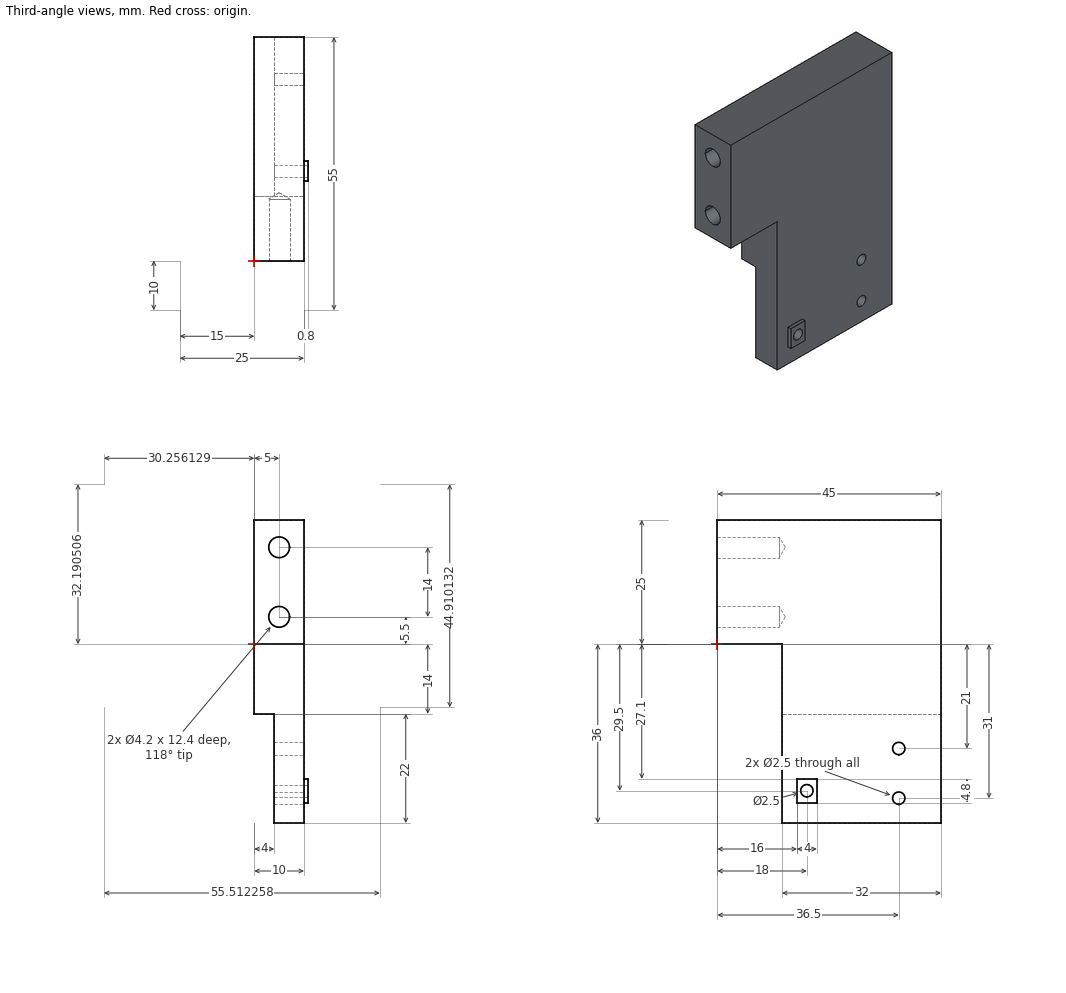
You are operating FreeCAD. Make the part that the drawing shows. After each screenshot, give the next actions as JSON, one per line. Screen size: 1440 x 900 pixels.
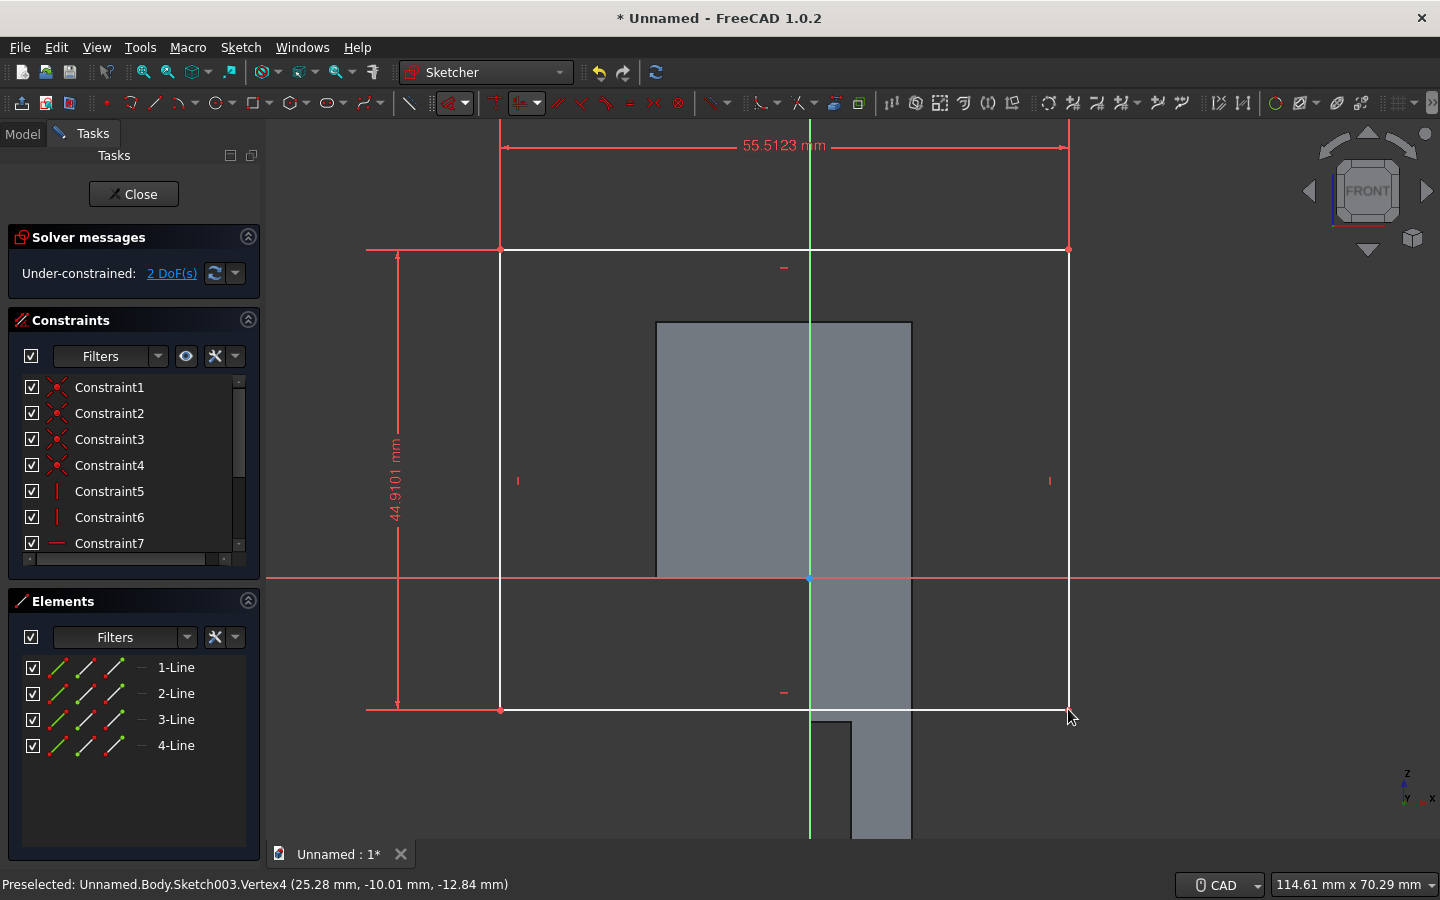
{"action": "left_click", "coordinate": [500, 250]}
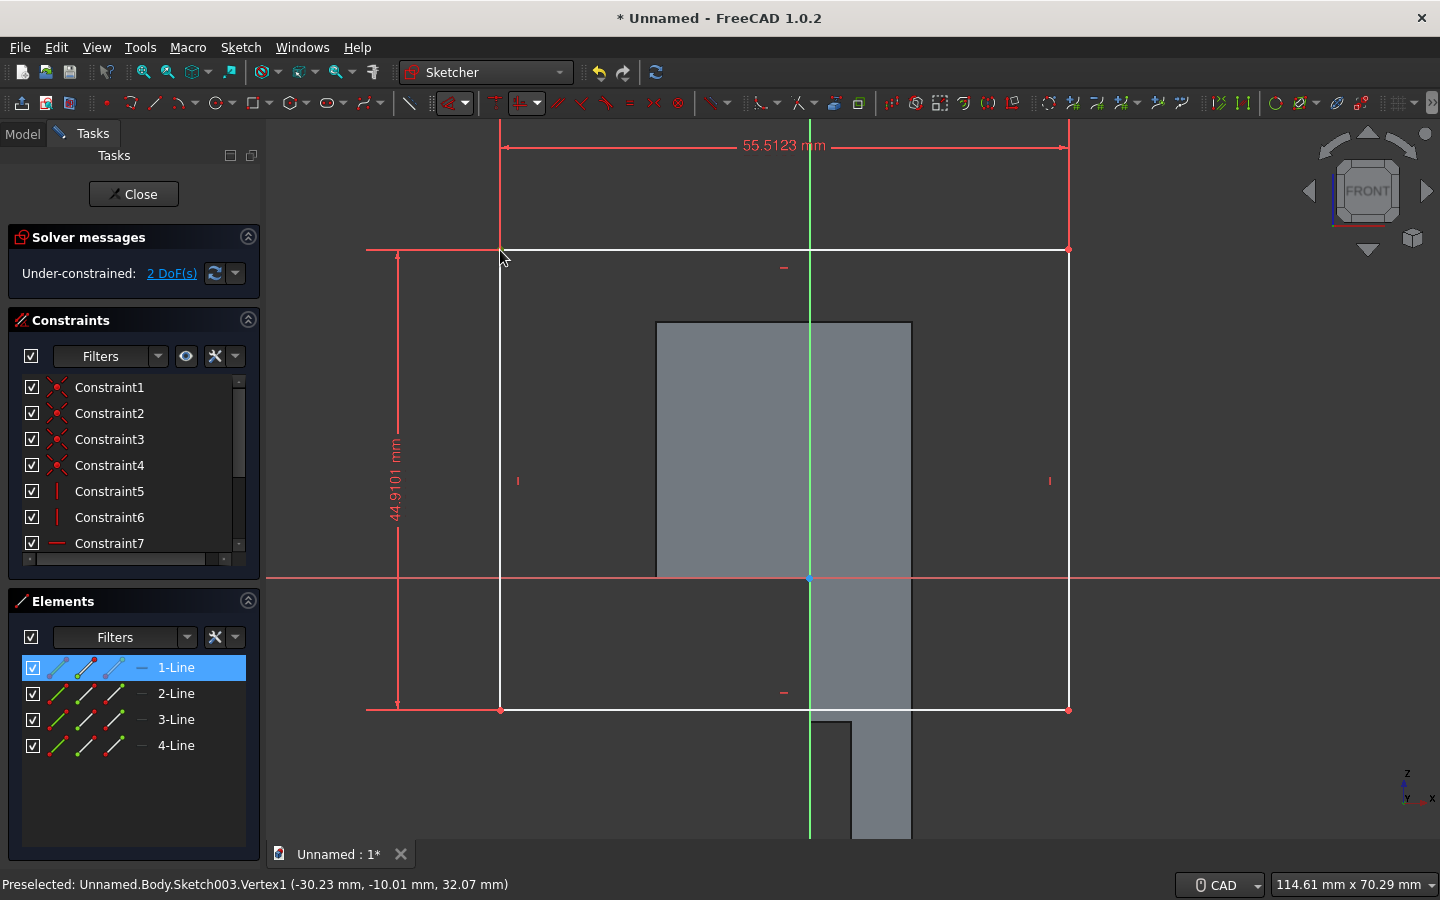
{"action": "key", "text": "l"}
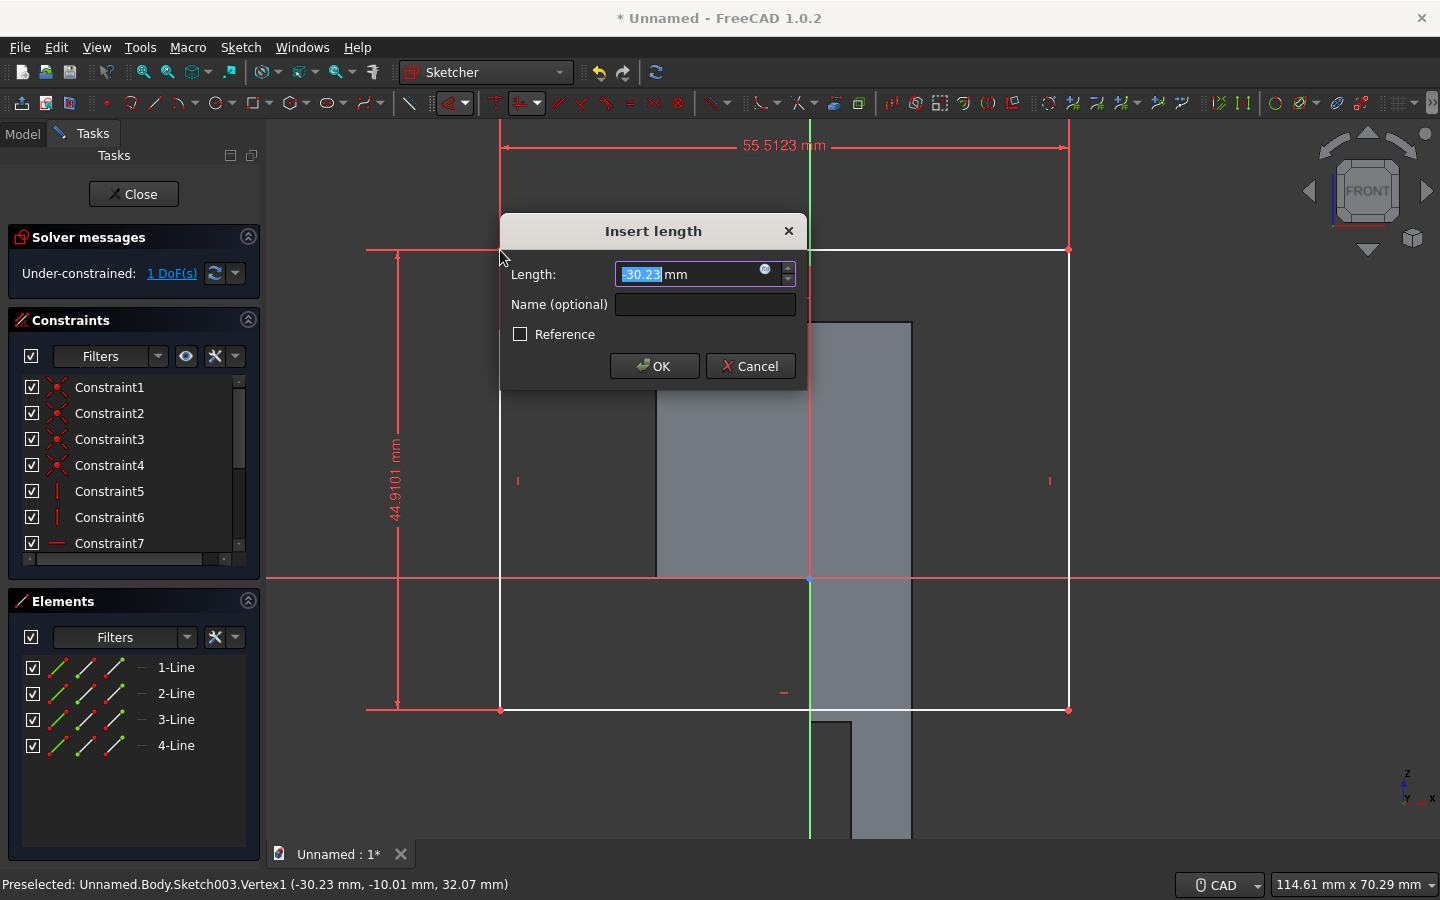
{"action": "type", "text": "-30.256129"}
{"action": "key", "text": "Return"}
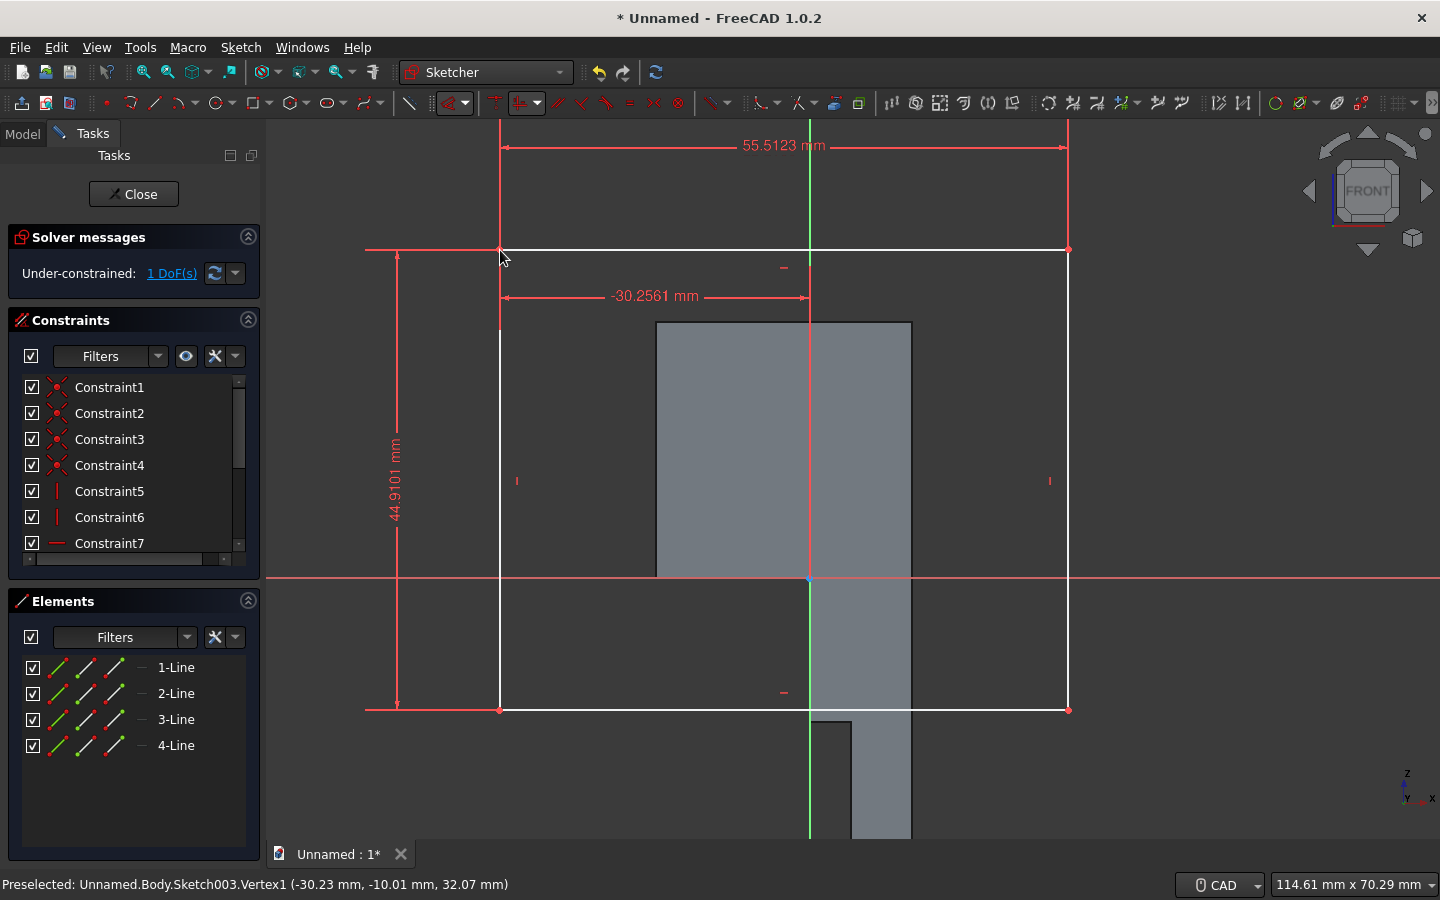
{"action": "left_click", "coordinate": [500, 250]}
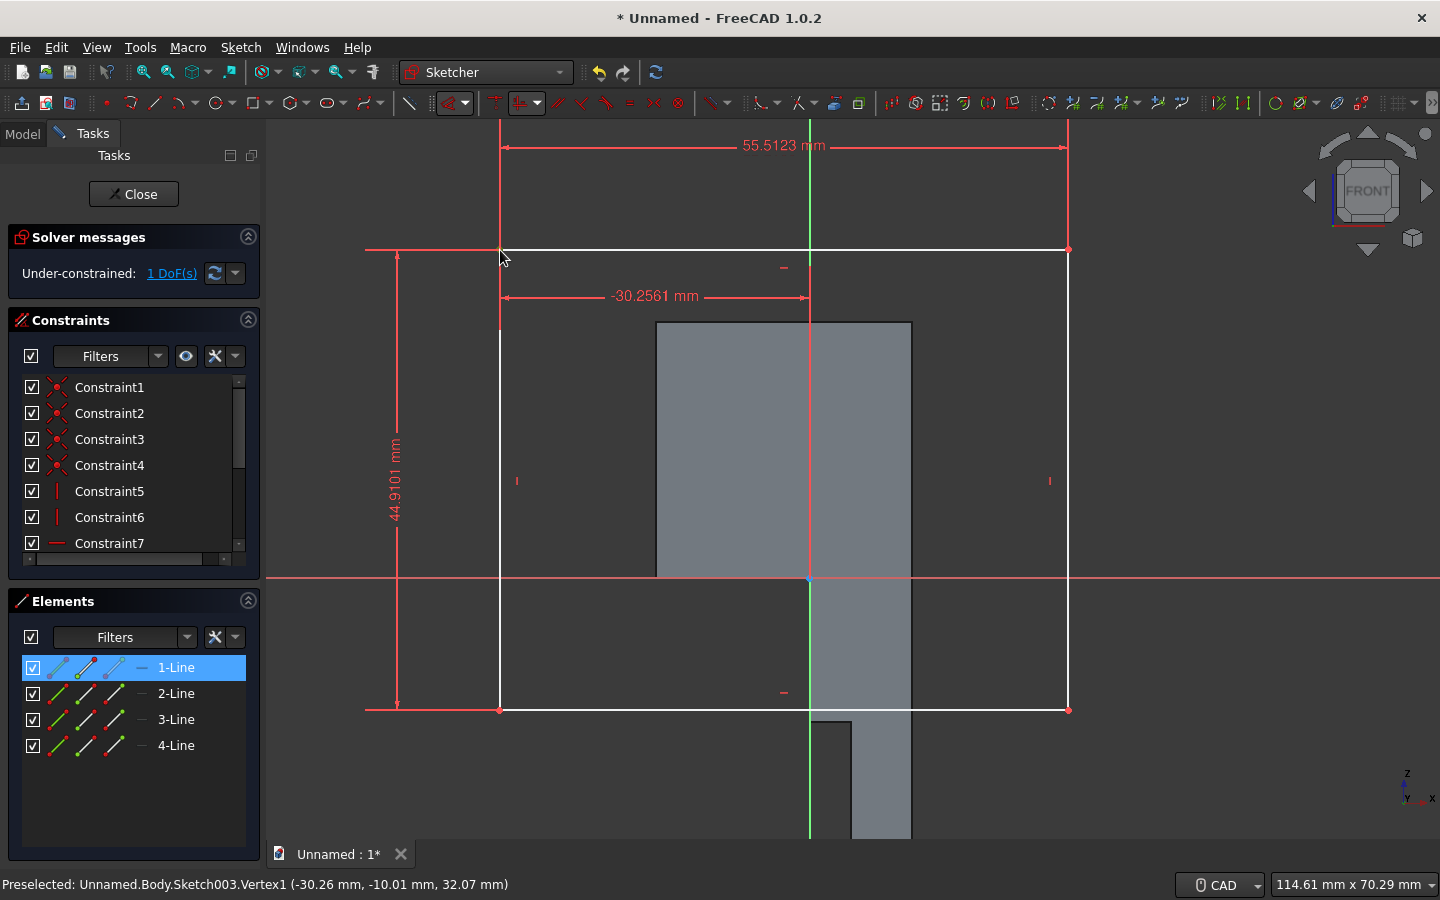
{"action": "key", "text": "i"}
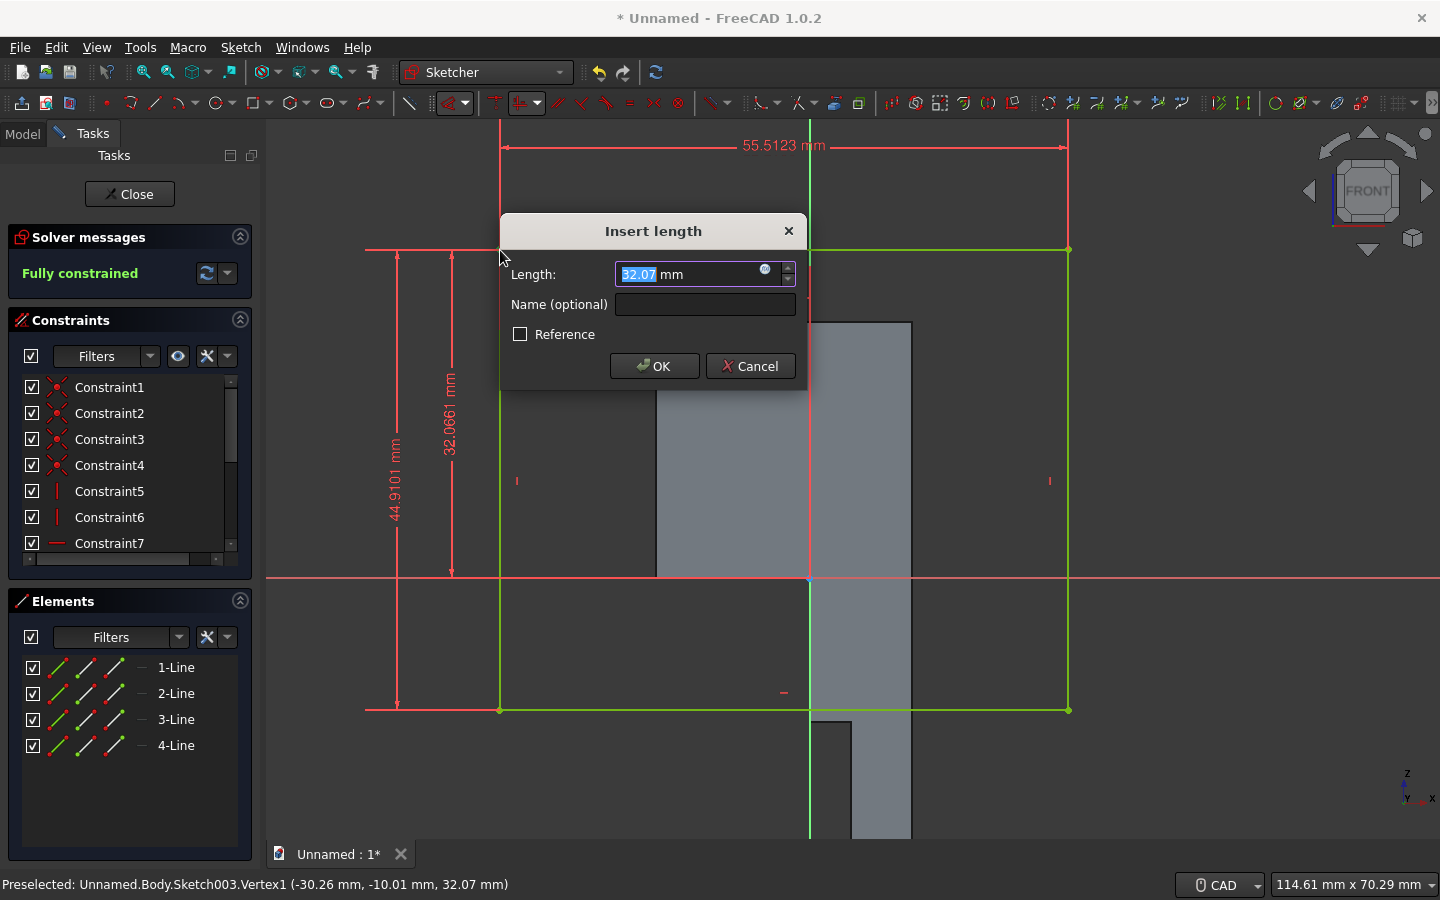
{"action": "type", "text": "32.190506"}
{"action": "key", "text": "Return"}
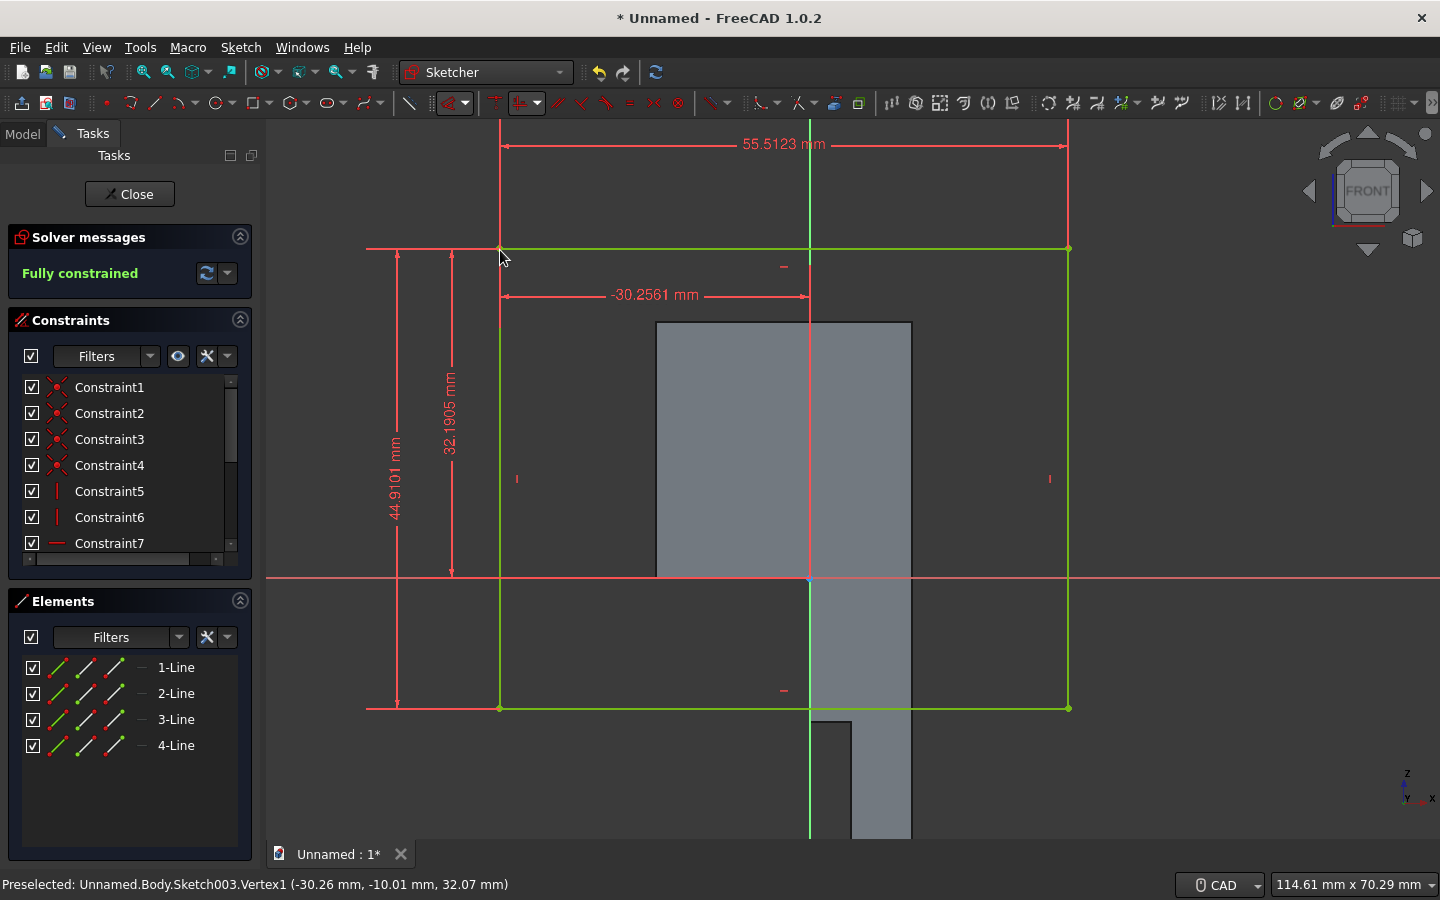
{"action": "left_click", "coordinate": [130, 194]}